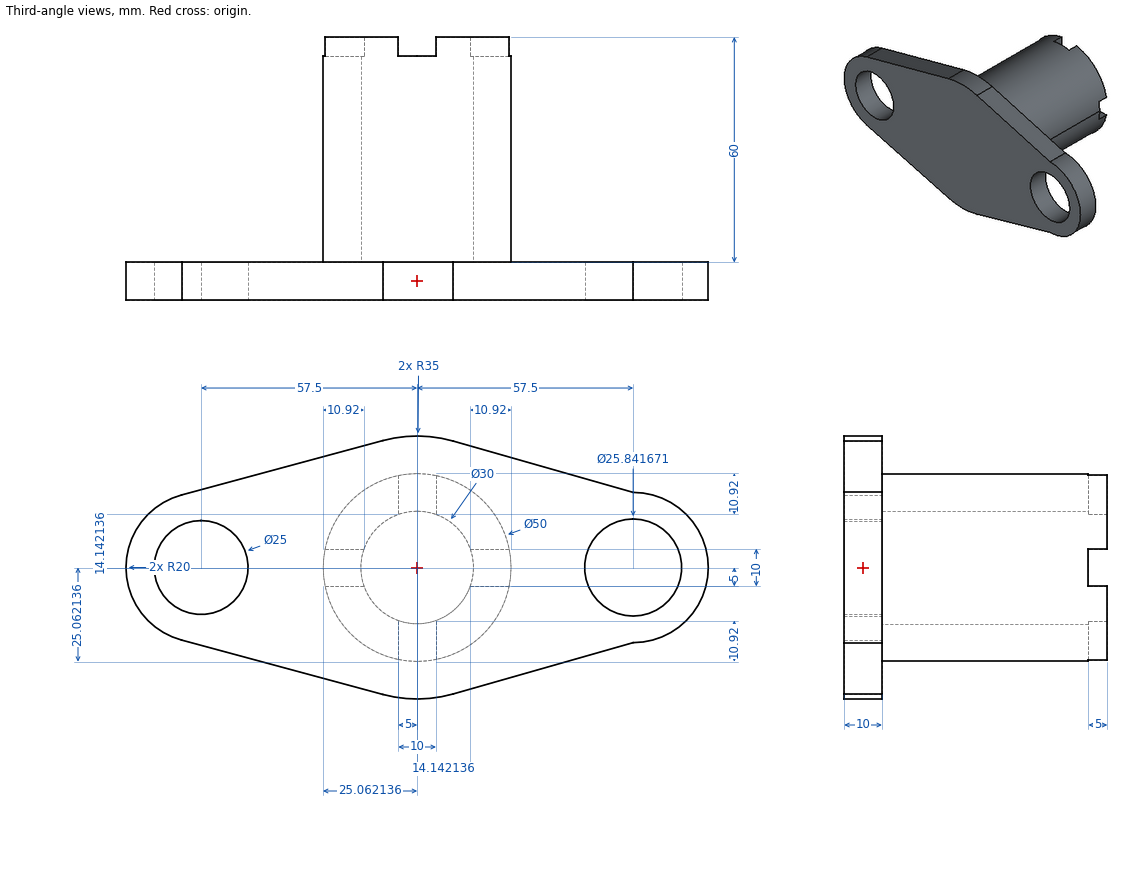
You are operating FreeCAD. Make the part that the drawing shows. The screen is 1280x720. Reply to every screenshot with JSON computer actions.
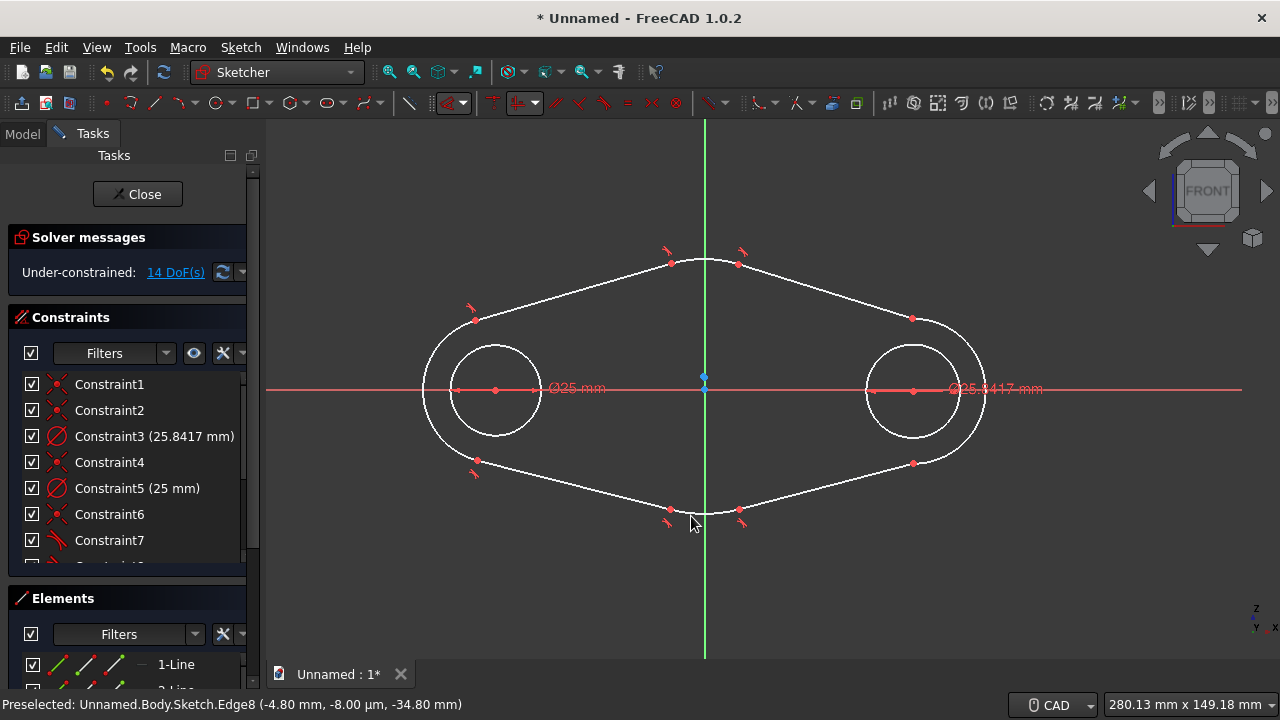
{"action": "left_click", "coordinate": [719, 260]}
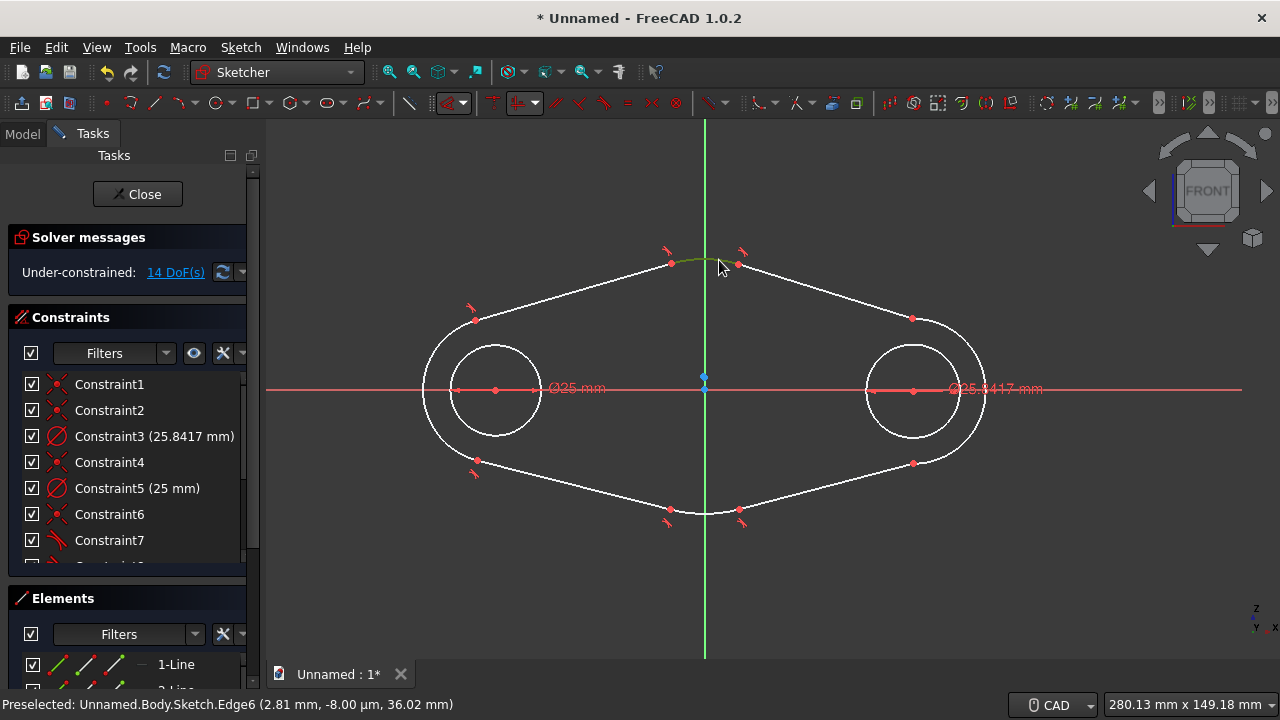
{"action": "left_click", "coordinate": [691, 513]}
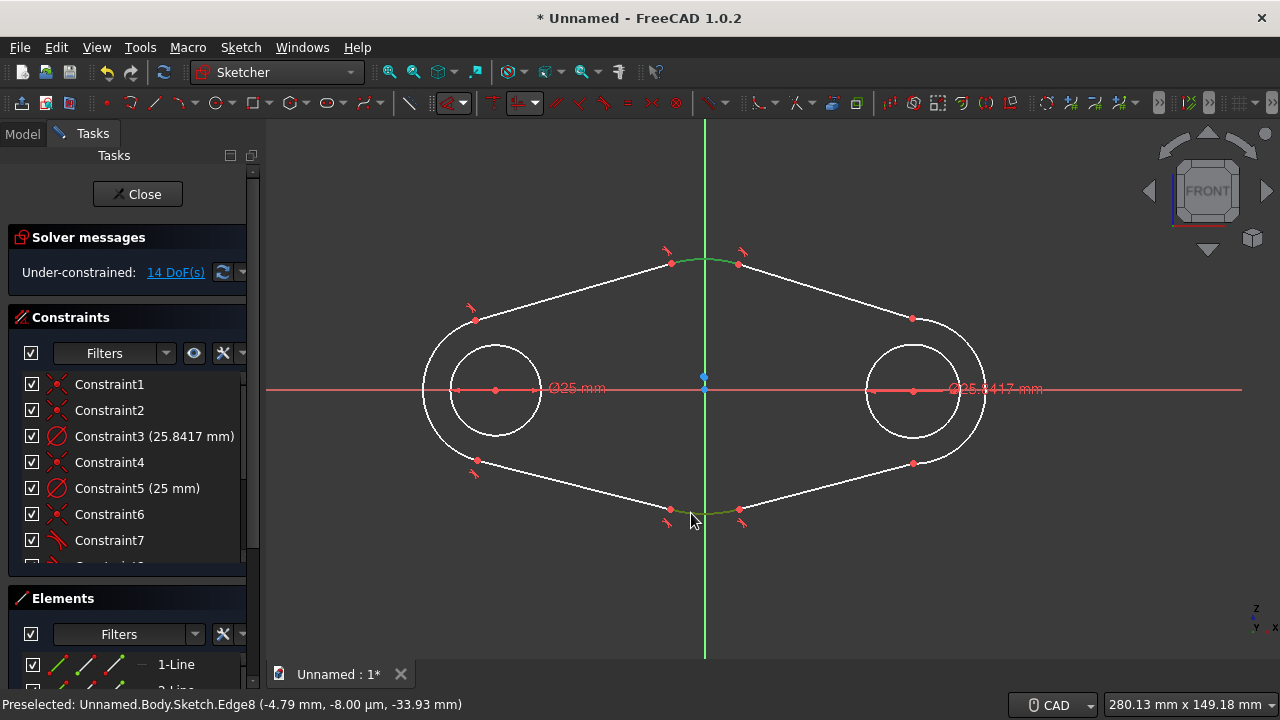
{"action": "key", "text": "c"}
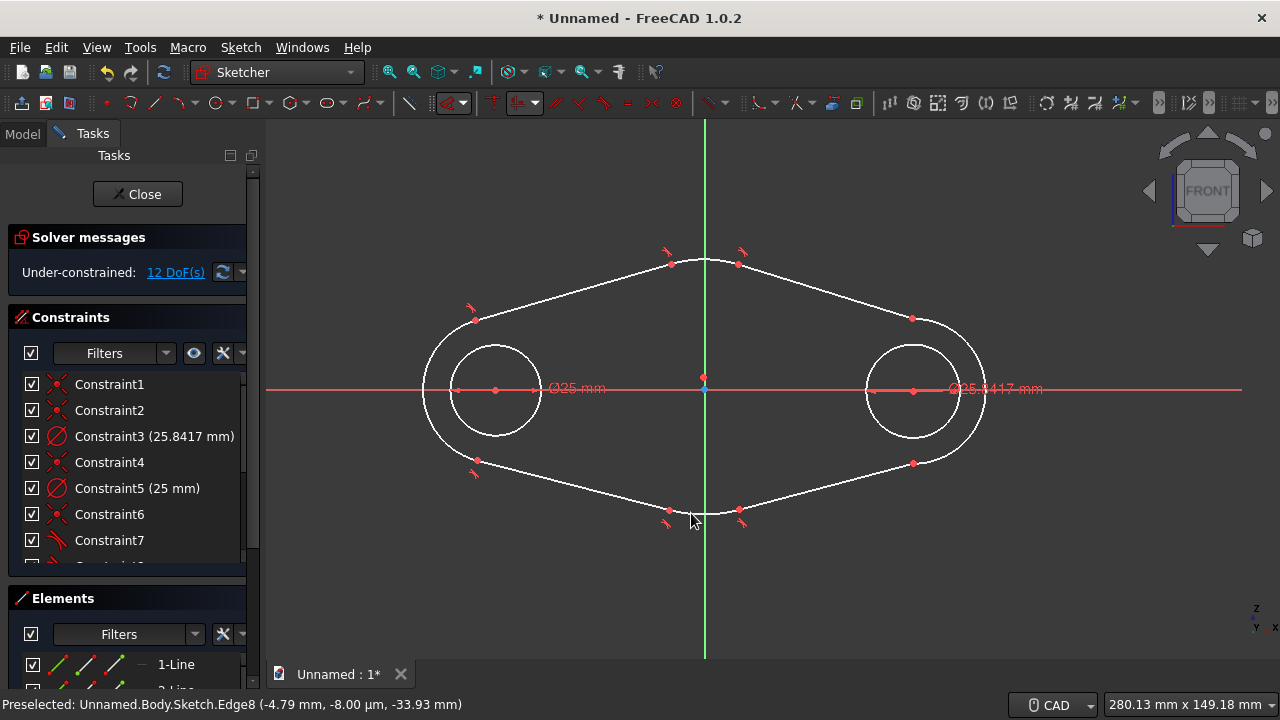
{"action": "left_click_drag", "start_coordinate": [694, 368], "coordinate": [715, 400]}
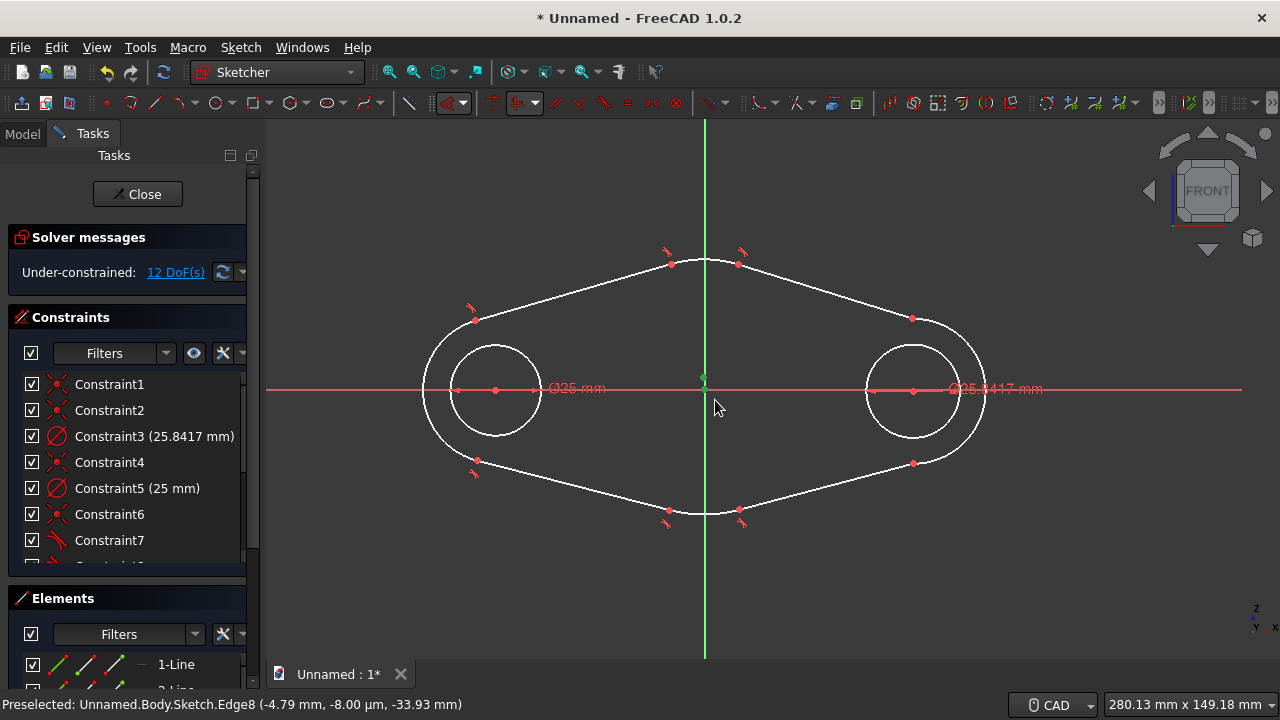
{"action": "key", "text": "c"}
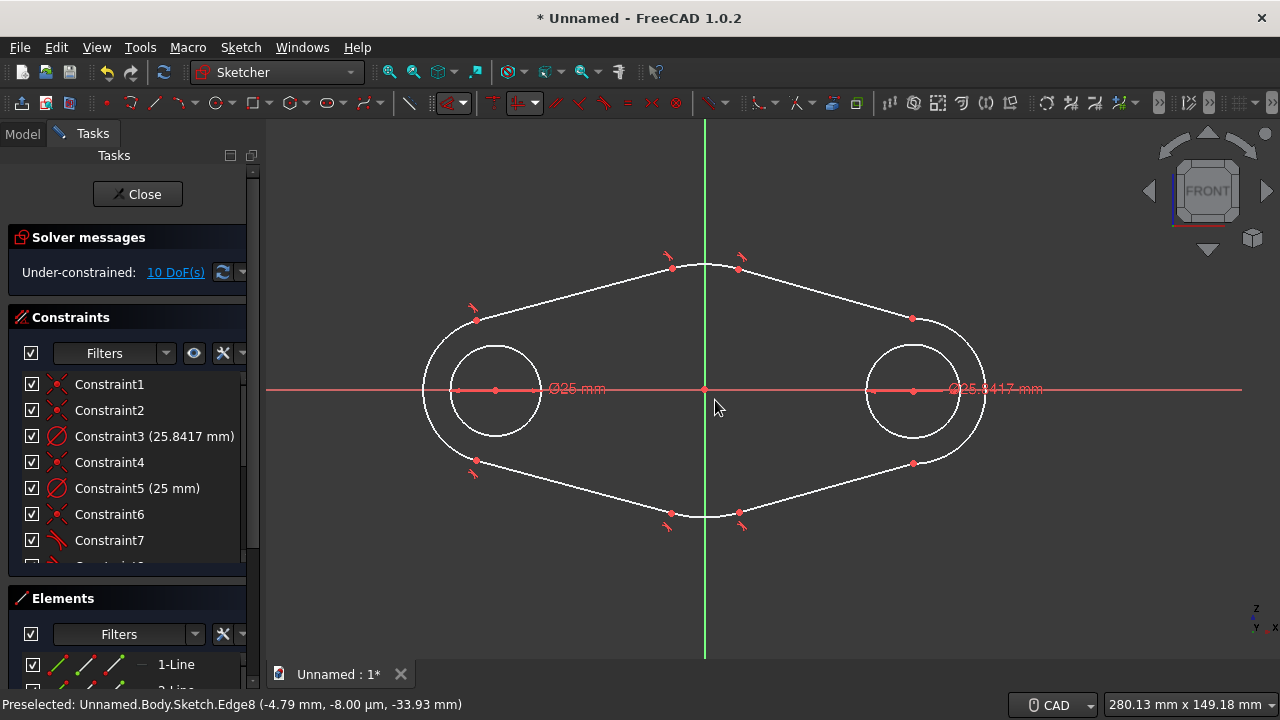
{"action": "left_click", "coordinate": [433, 355]}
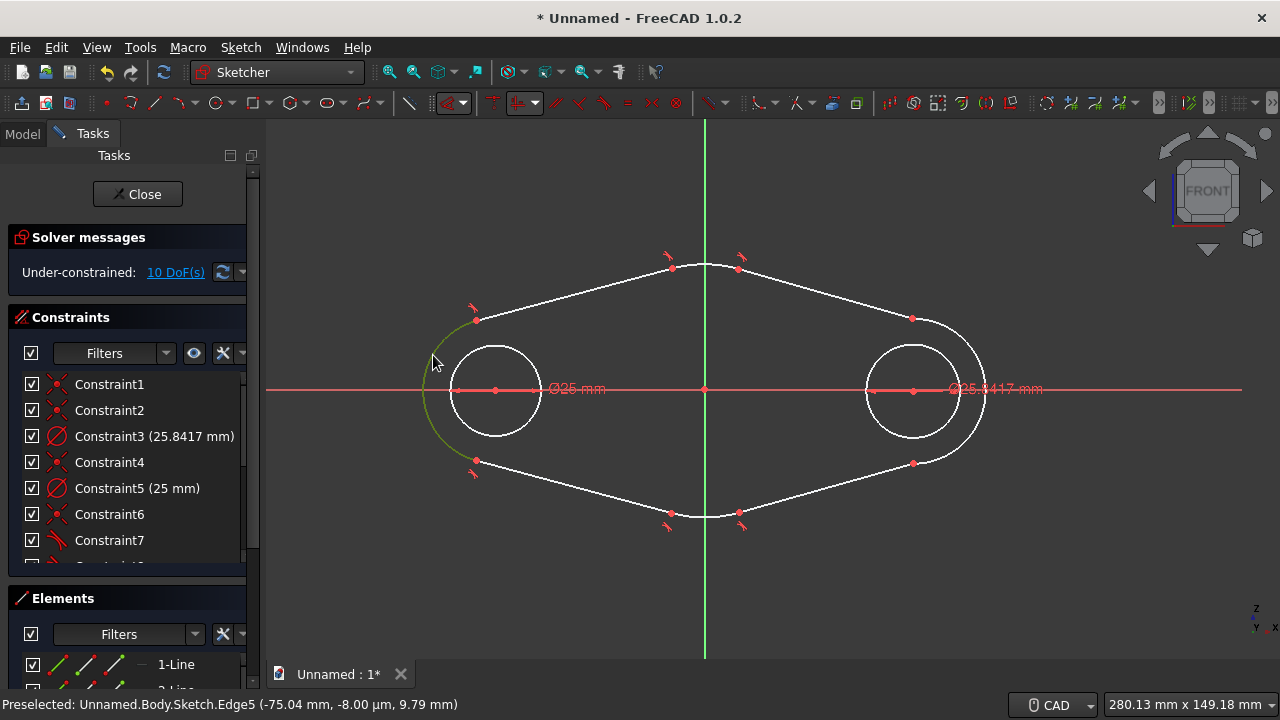
{"action": "left_click", "coordinate": [972, 434]}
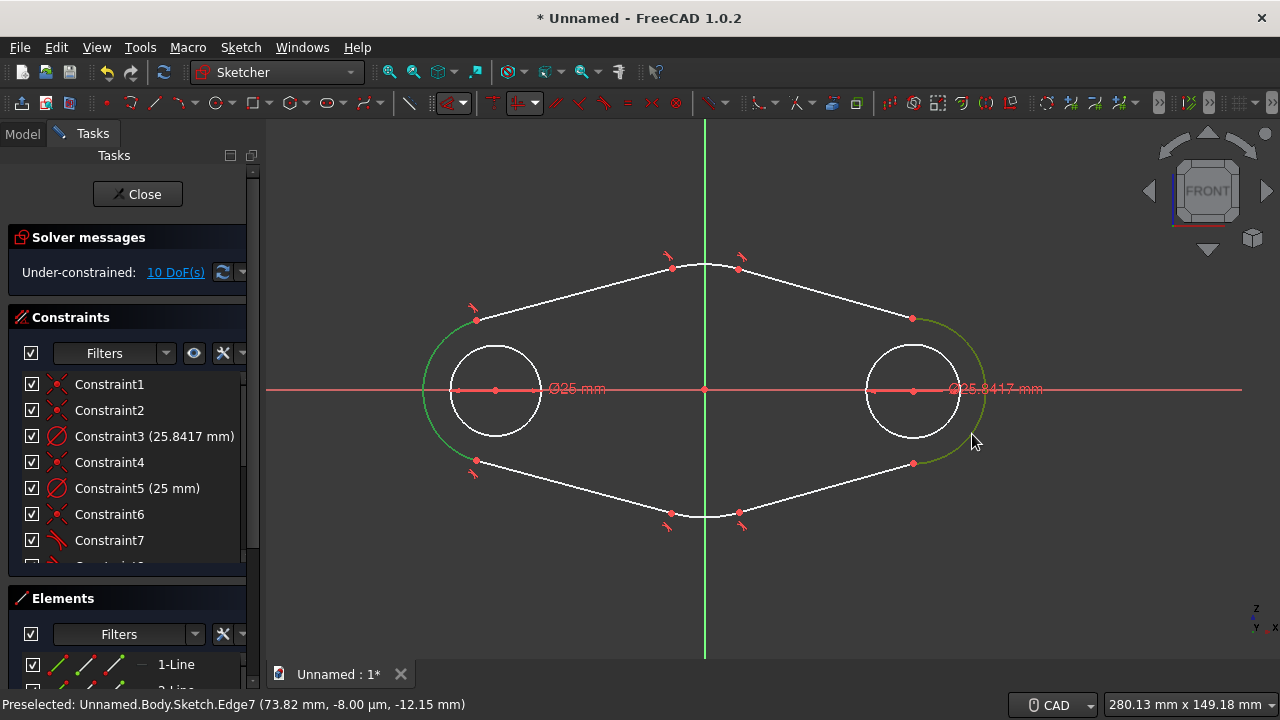
{"action": "key", "text": "e"}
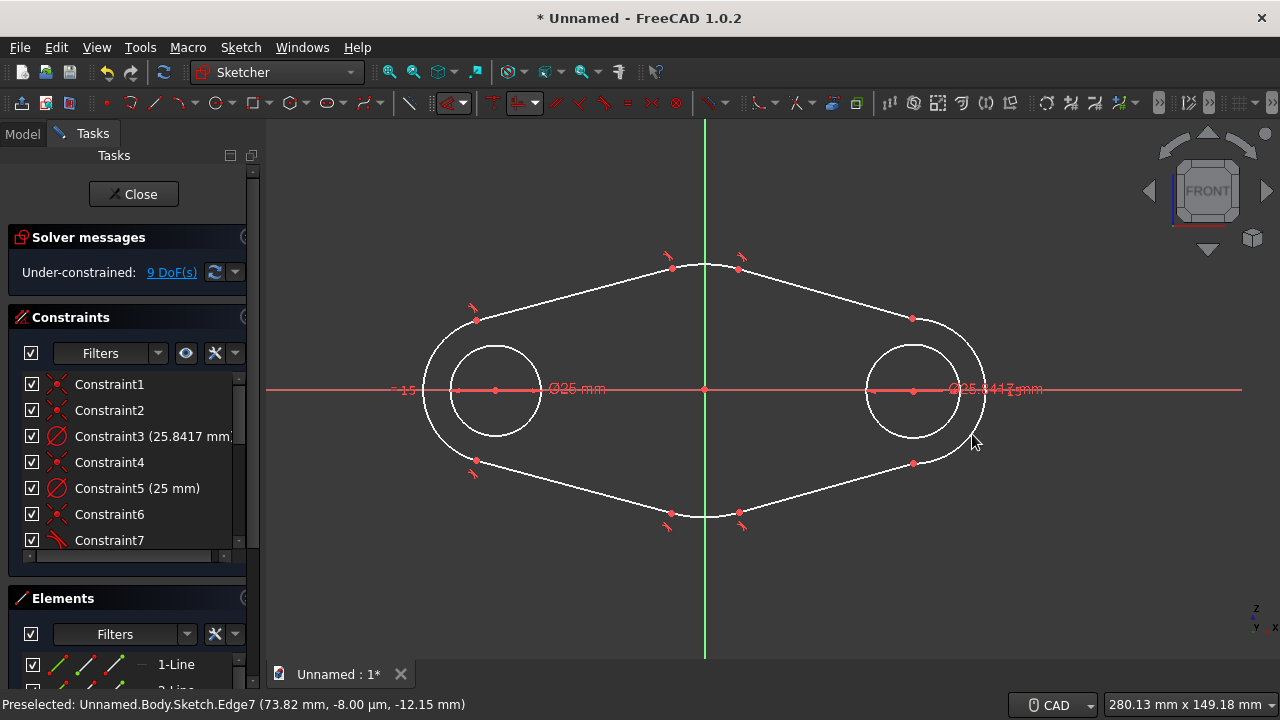
{"action": "left_click", "coordinate": [719, 265]}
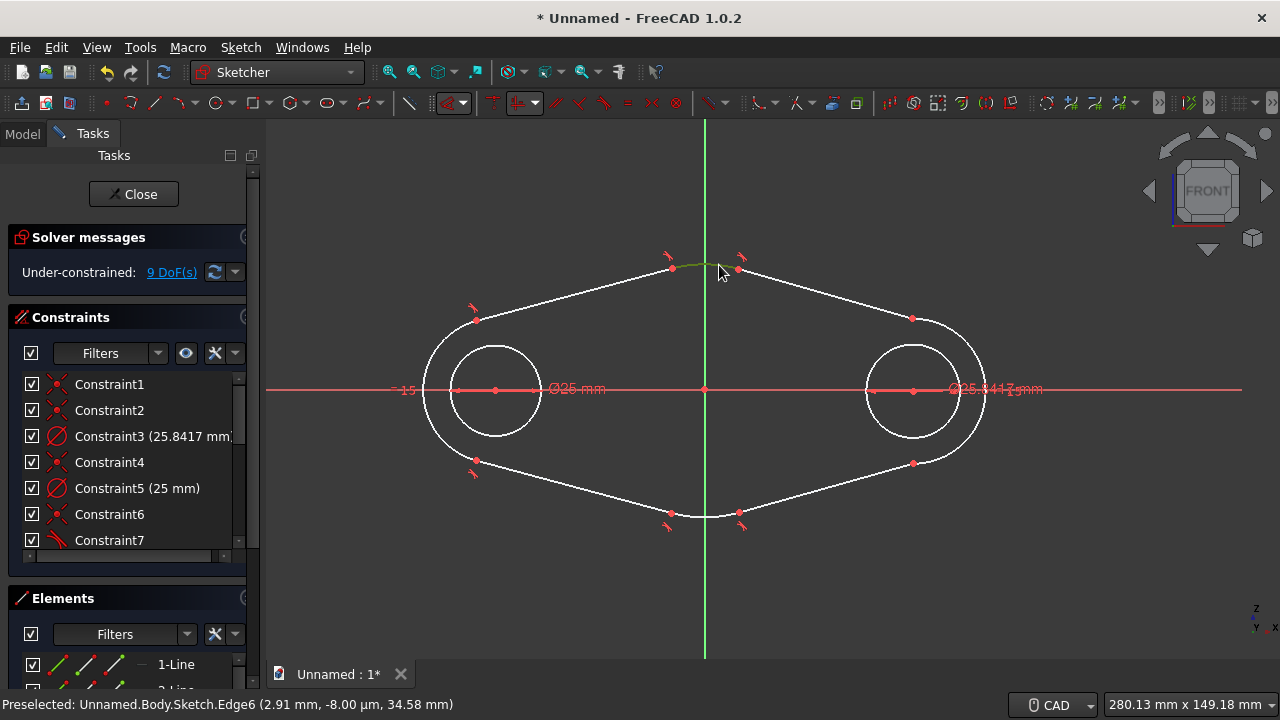
{"action": "left_click", "coordinate": [692, 517]}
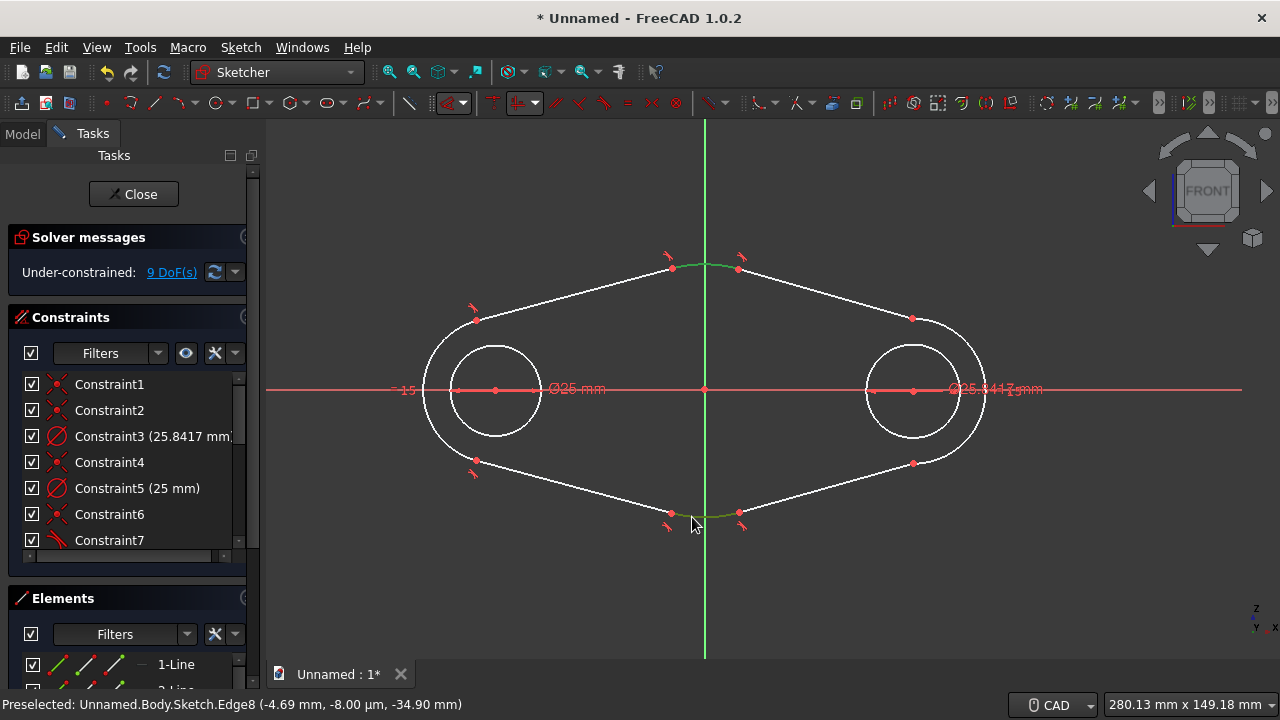
{"action": "key", "text": "e"}